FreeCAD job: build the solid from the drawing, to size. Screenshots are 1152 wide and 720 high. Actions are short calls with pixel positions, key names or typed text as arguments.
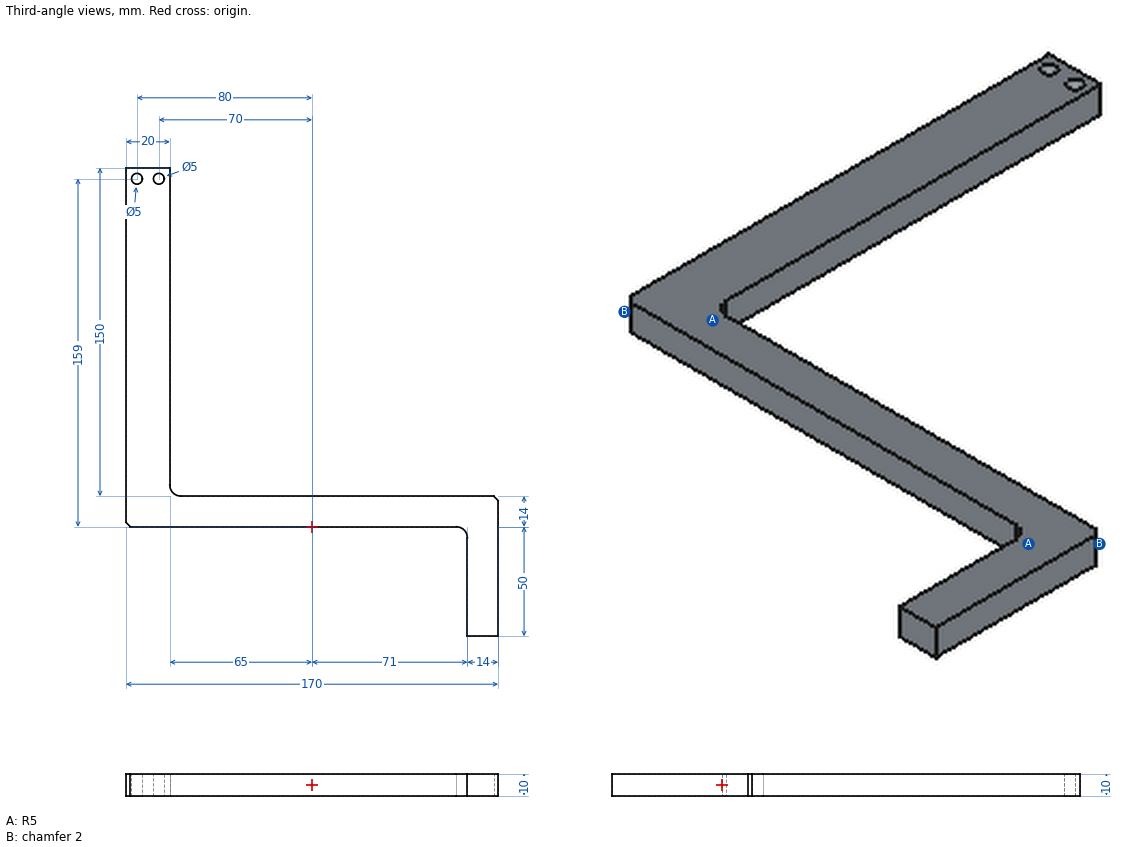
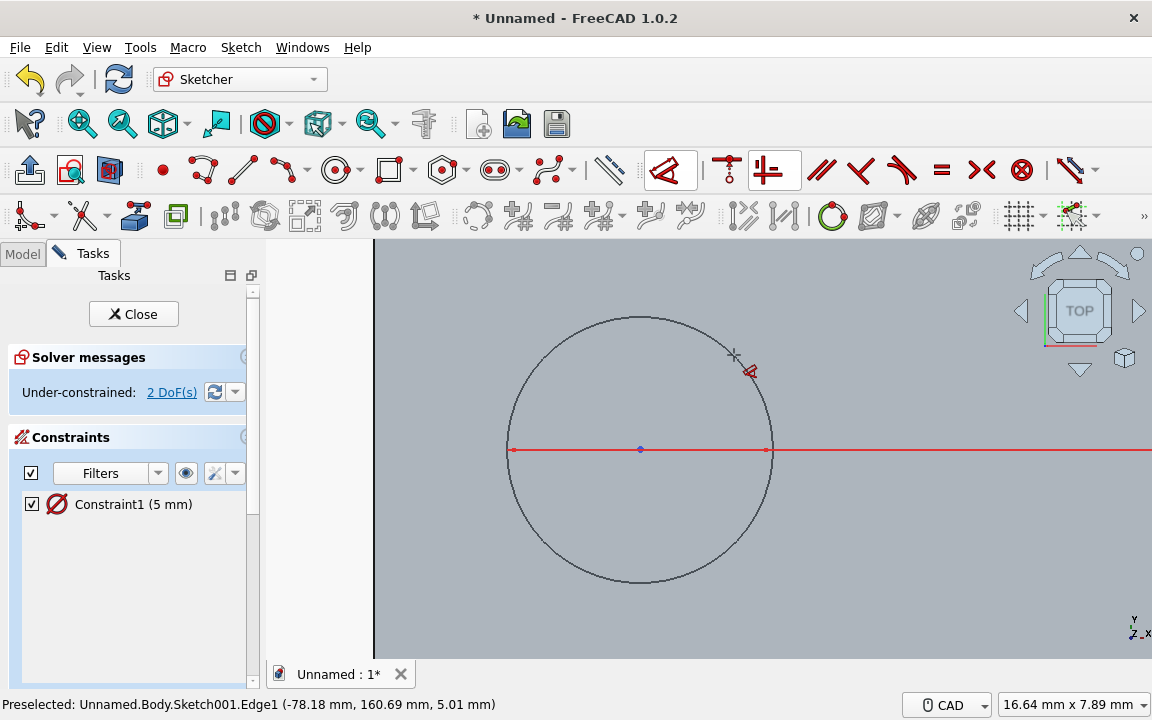
click(640, 450)
click(814, 416)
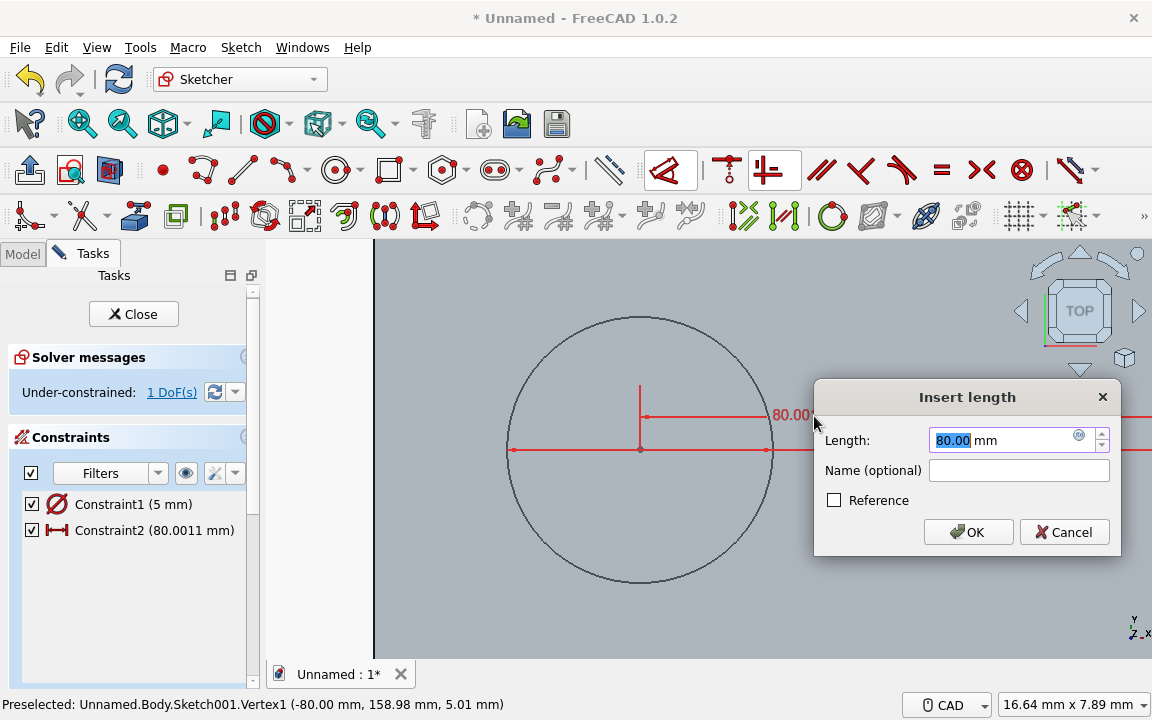
text(80)
key(Return)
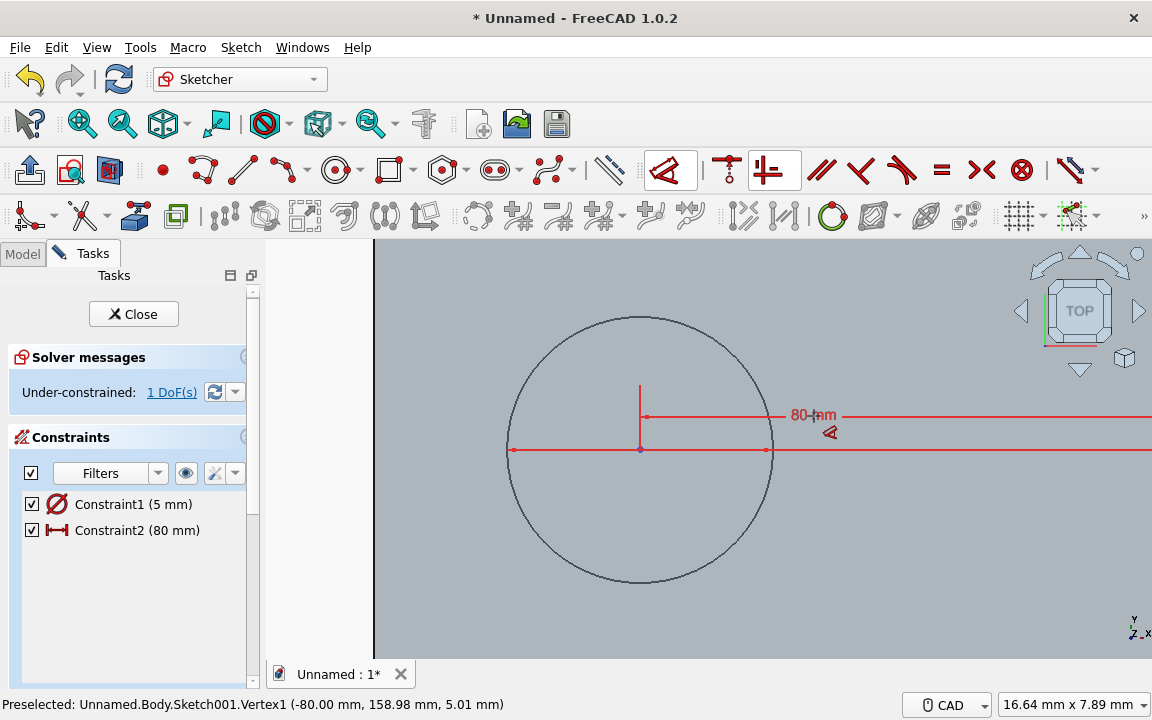
click(640, 450)
click(606, 540)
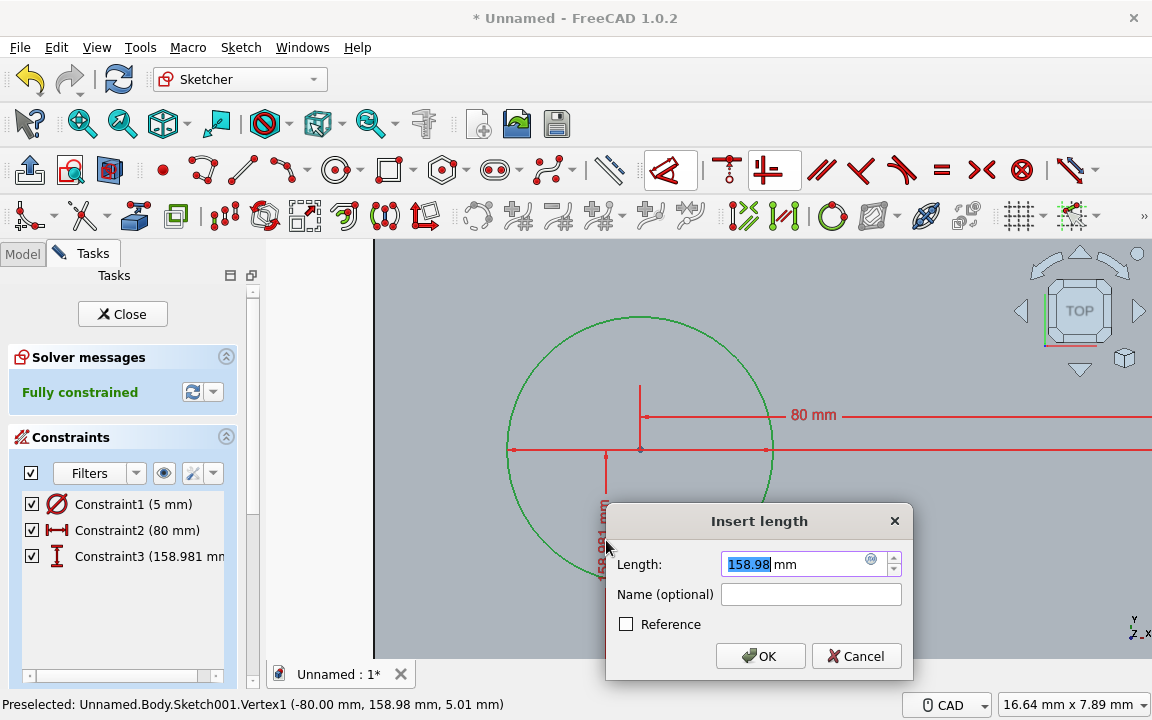
text(159)
key(Return)
key(Escape)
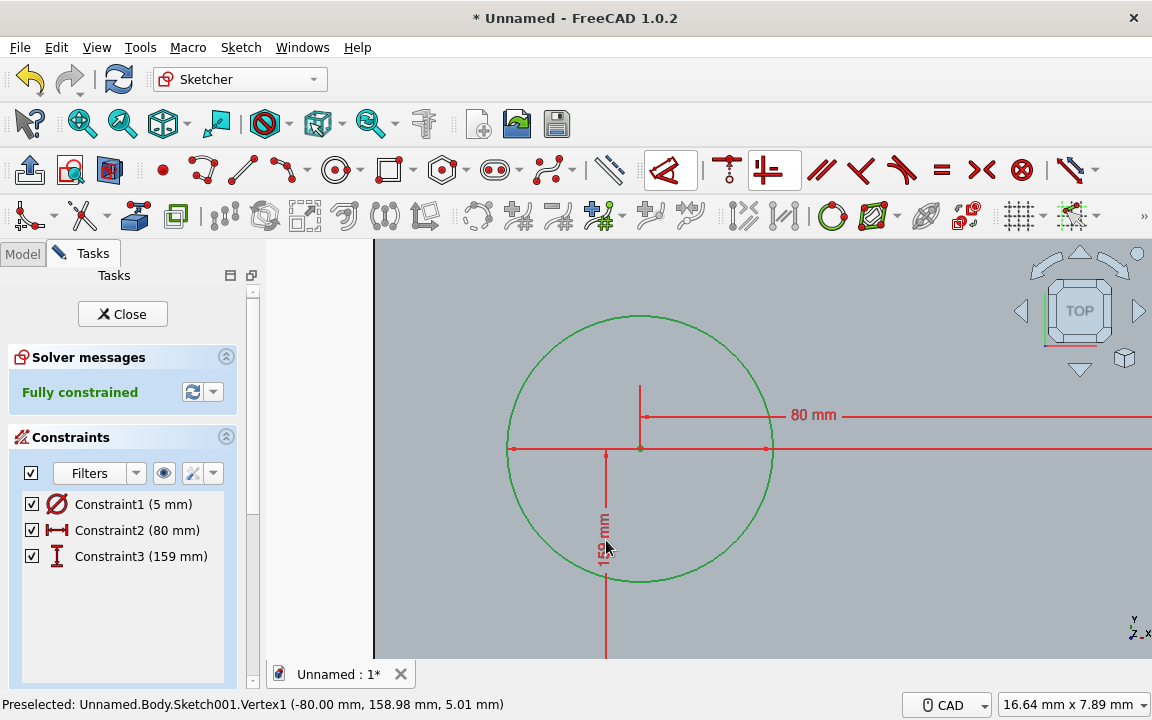
click(123, 314)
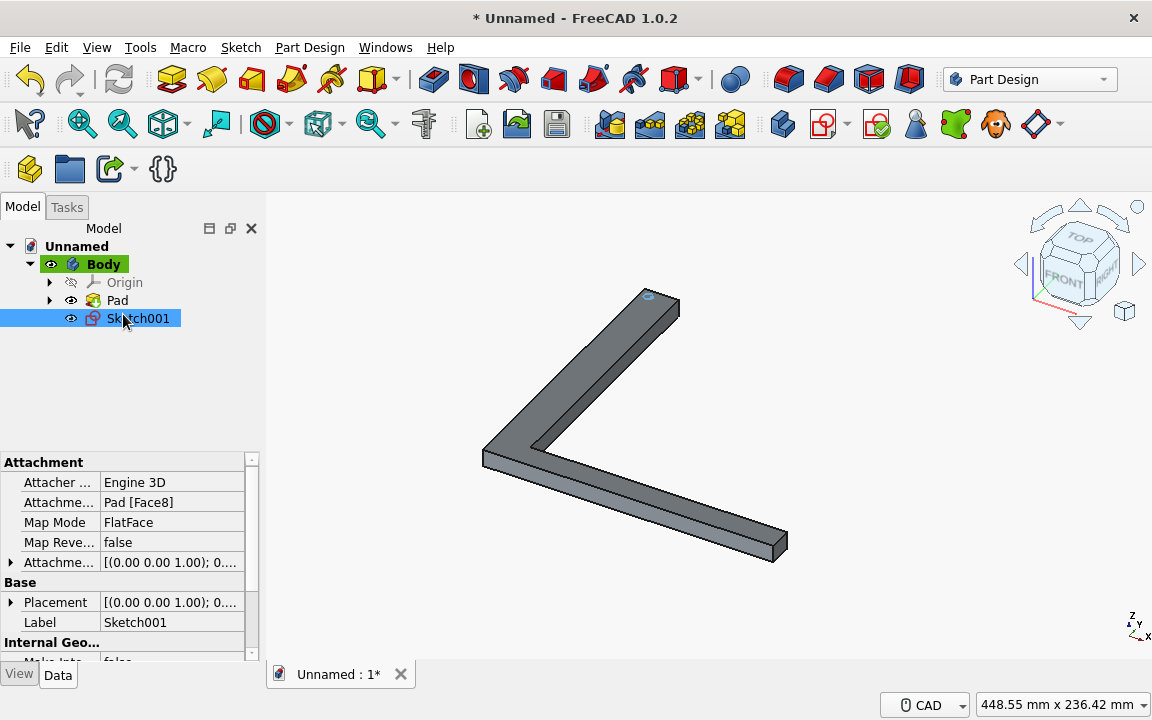
click(434, 80)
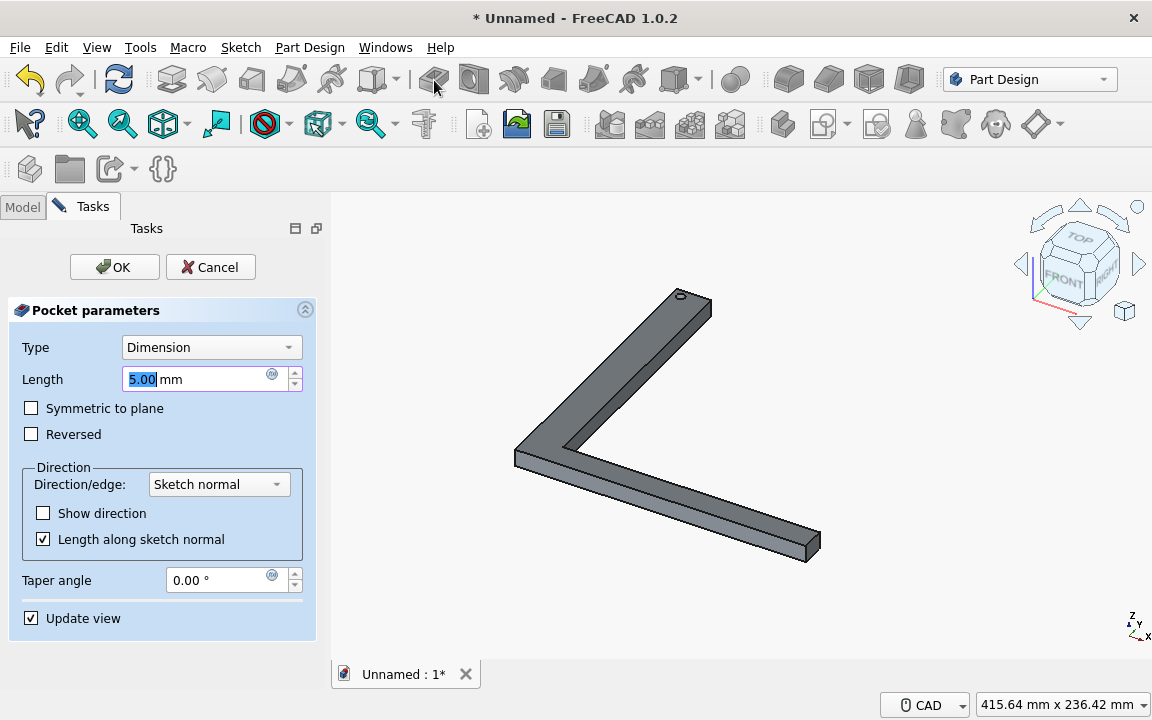
click(212, 348)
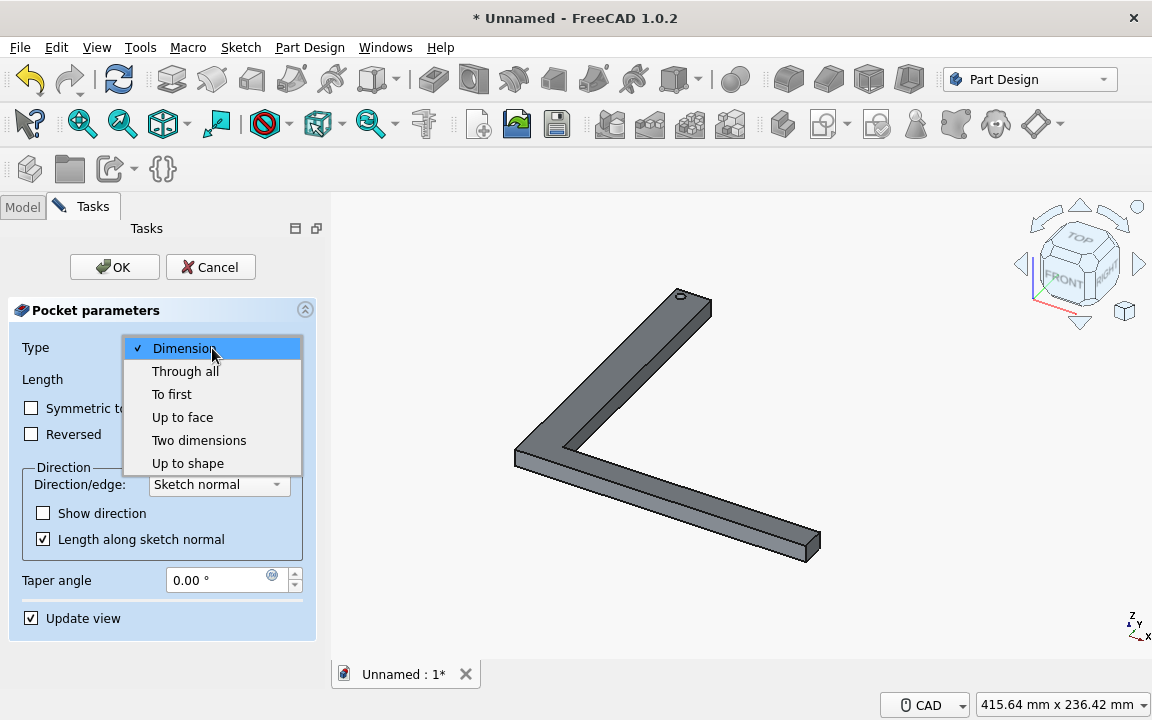
click(212, 394)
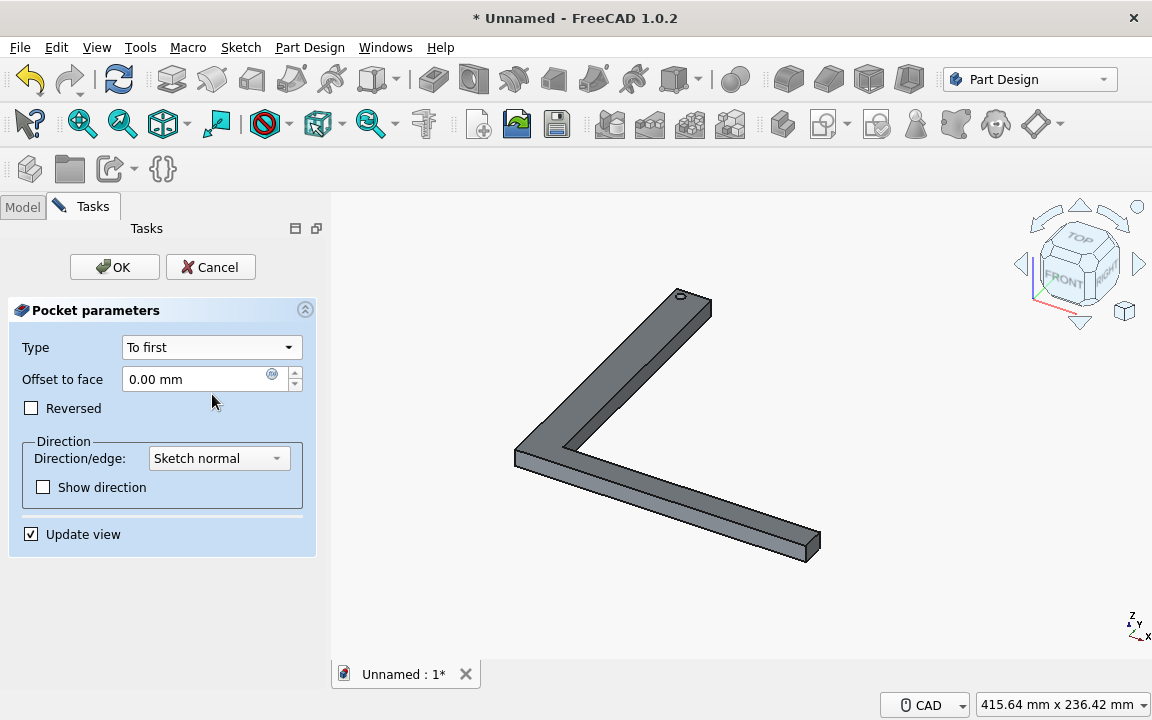
click(115, 267)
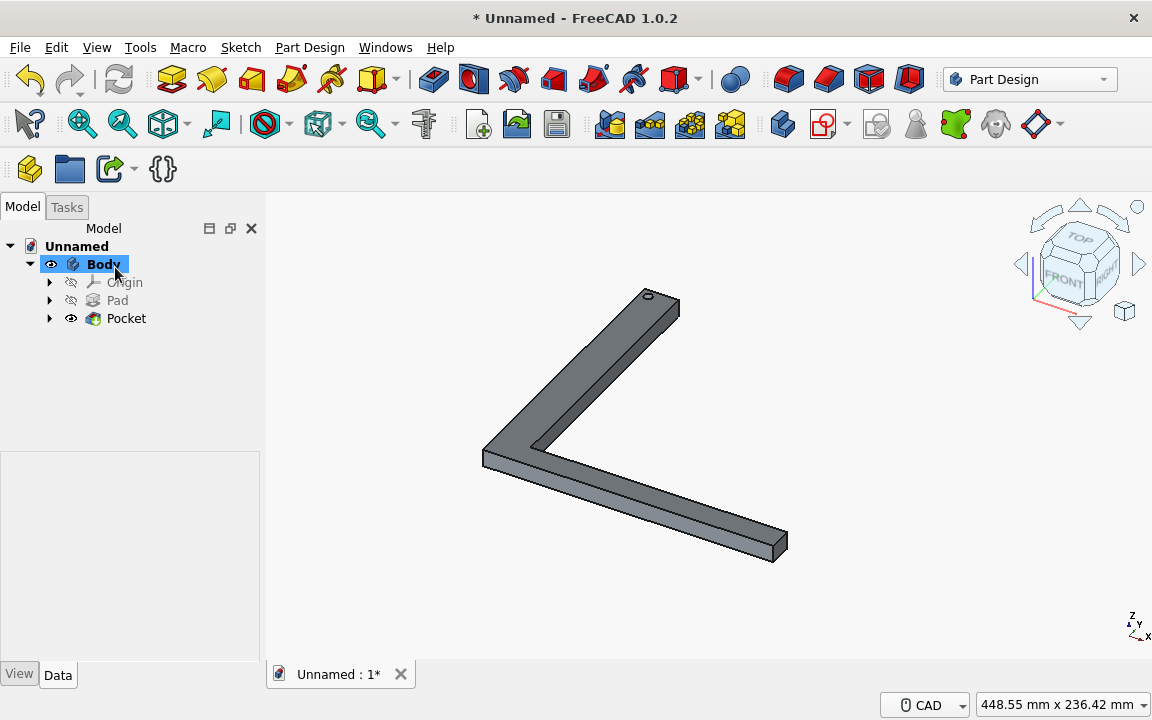
click(515, 444)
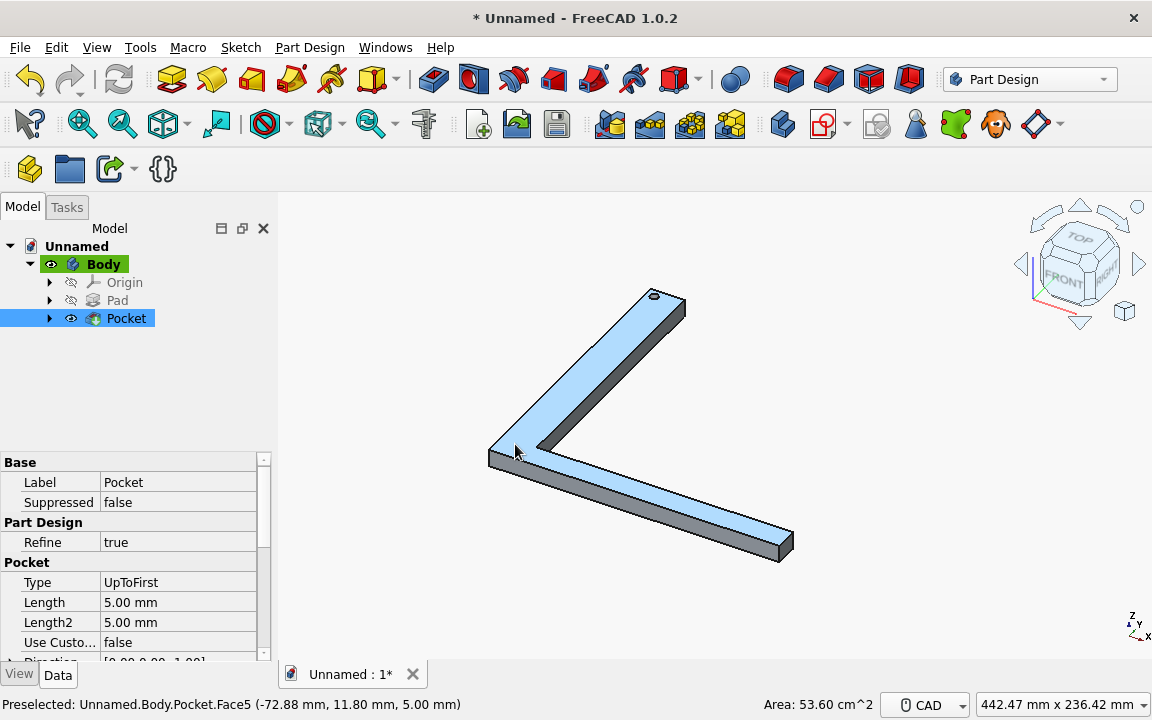
click(824, 124)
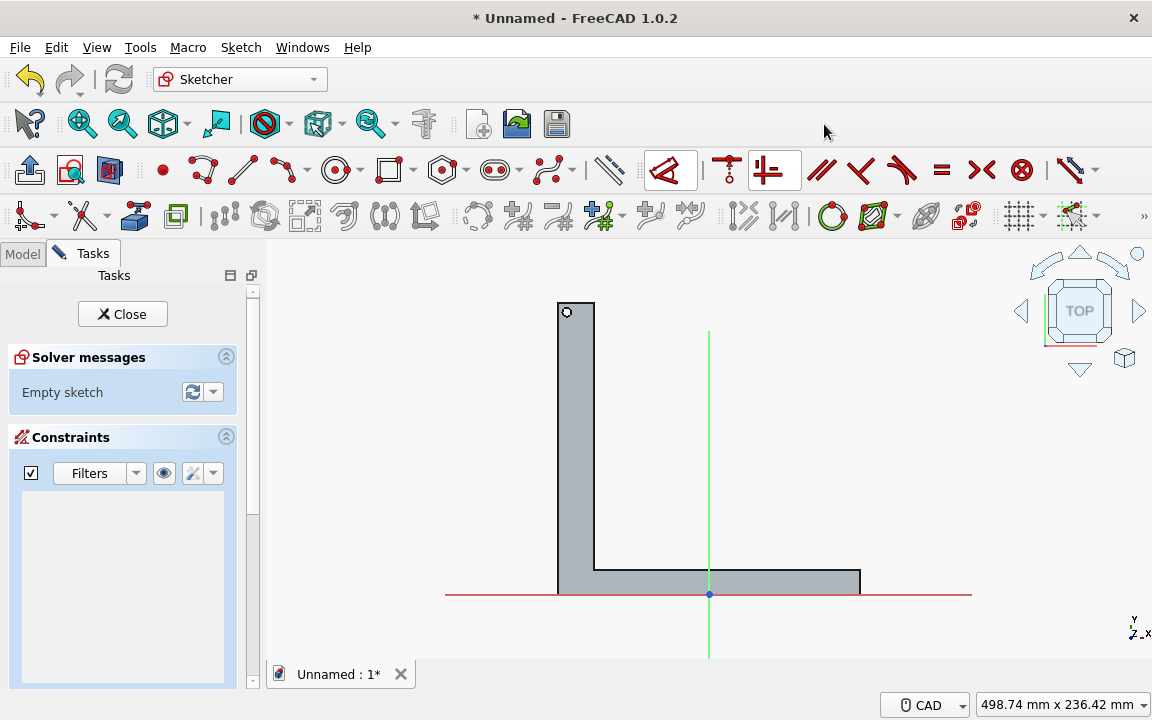
scroll(582, 305, up, 15)